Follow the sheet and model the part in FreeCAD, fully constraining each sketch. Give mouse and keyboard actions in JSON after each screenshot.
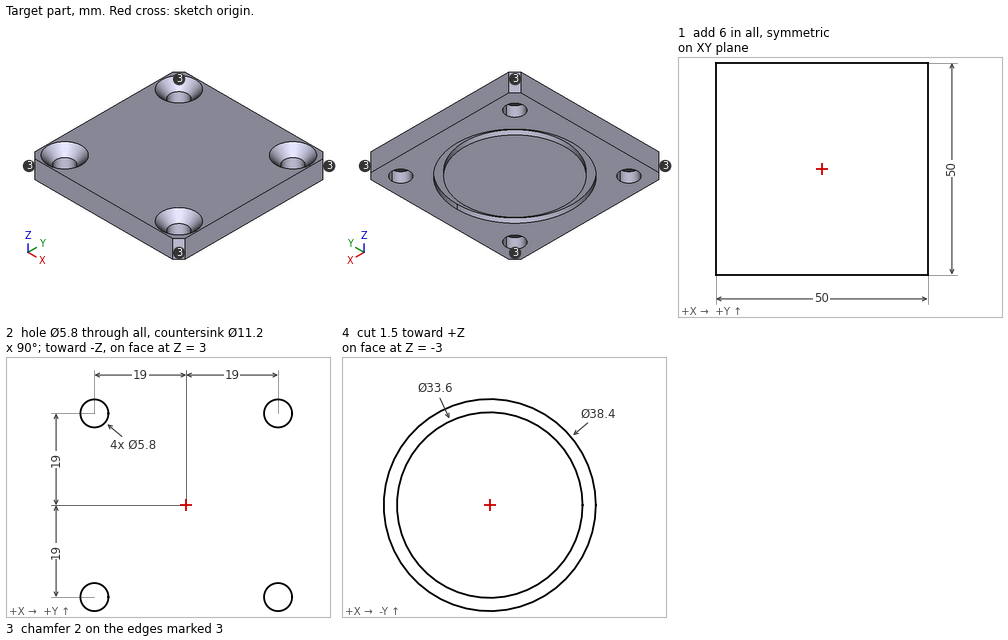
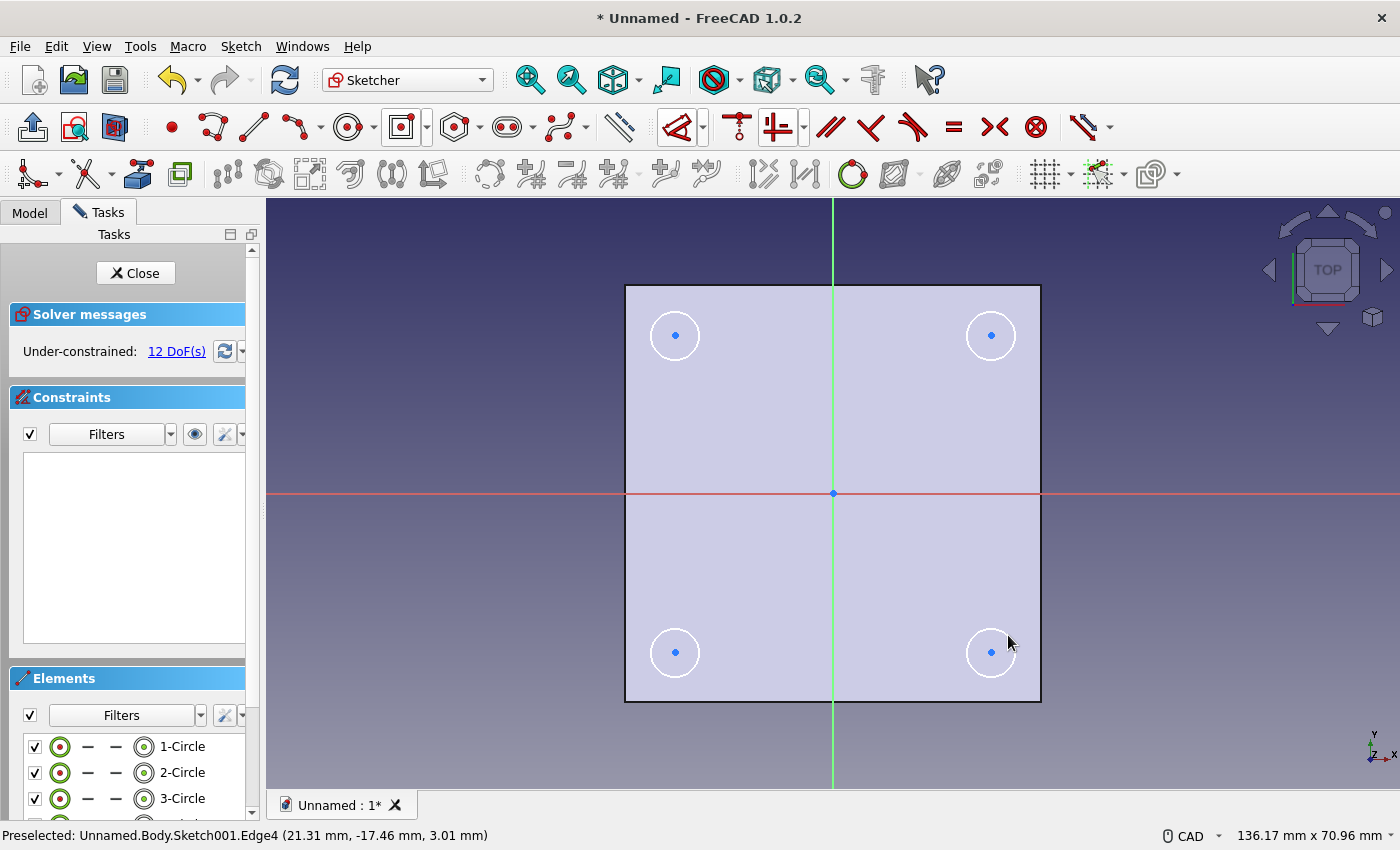
{"action": "left_click", "coordinate": [692, 319]}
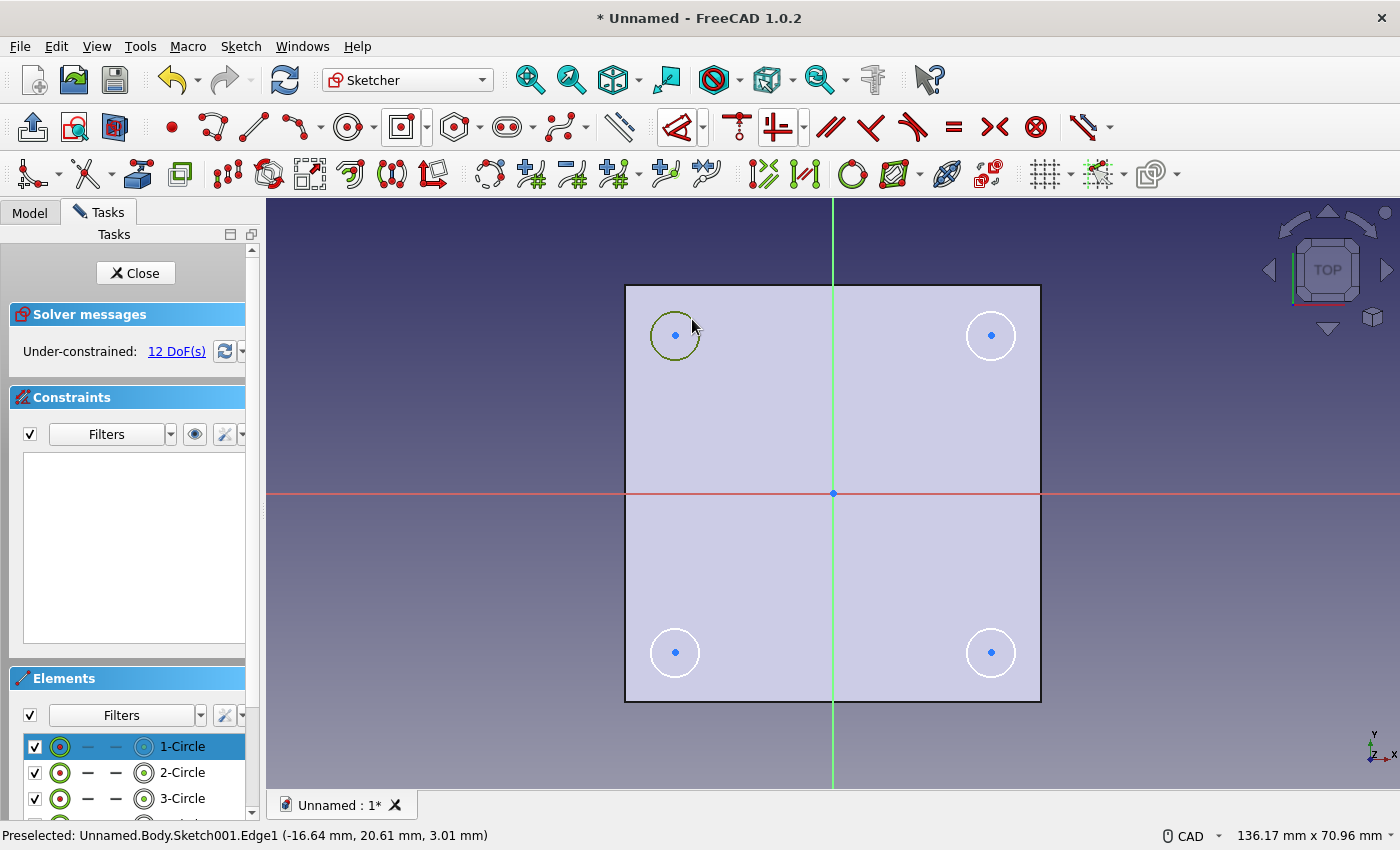
{"action": "left_click", "coordinate": [1008, 319]}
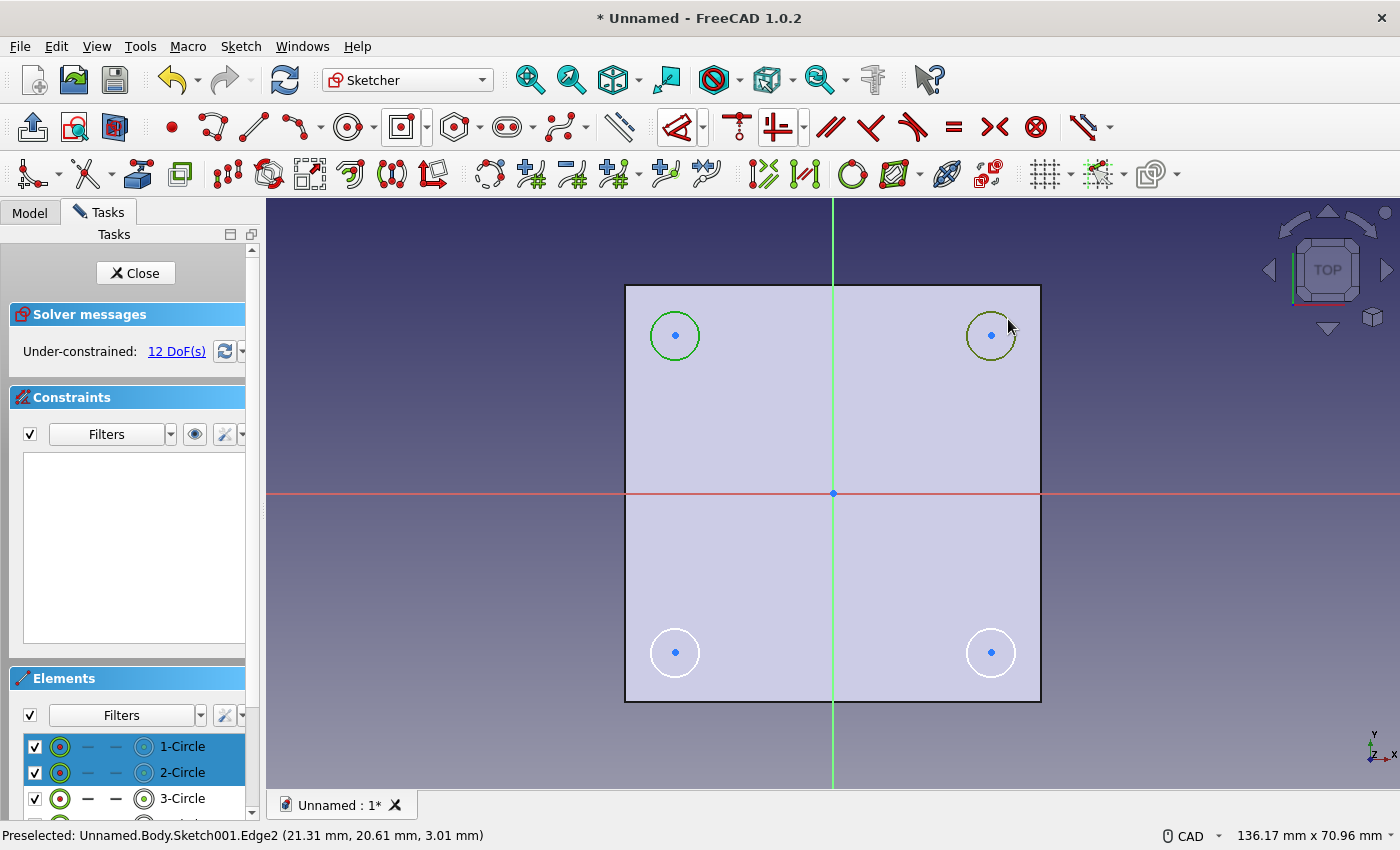
{"action": "left_click", "coordinate": [692, 636]}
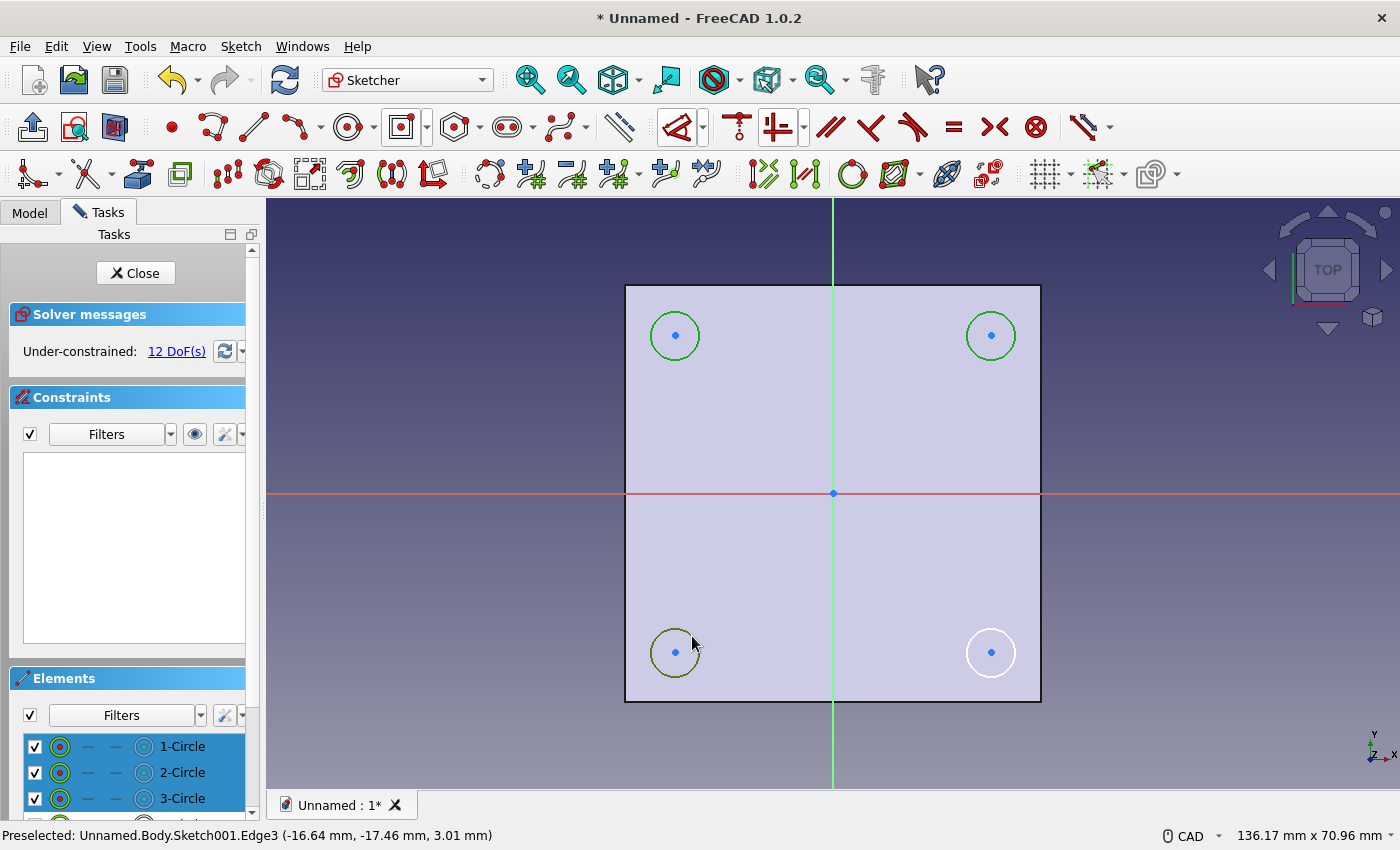
{"action": "left_click", "coordinate": [1008, 636]}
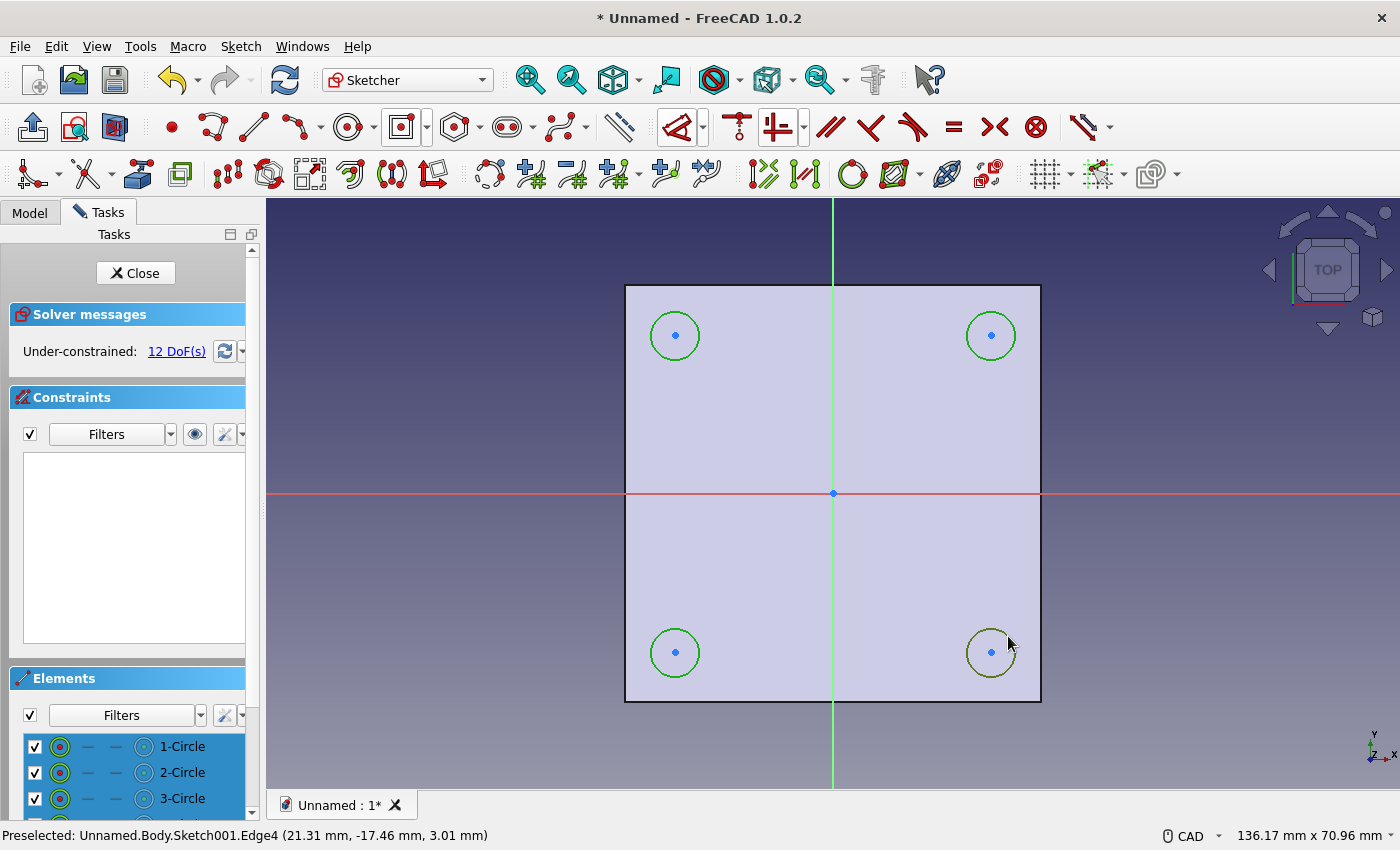
{"action": "left_click", "coordinate": [954, 128]}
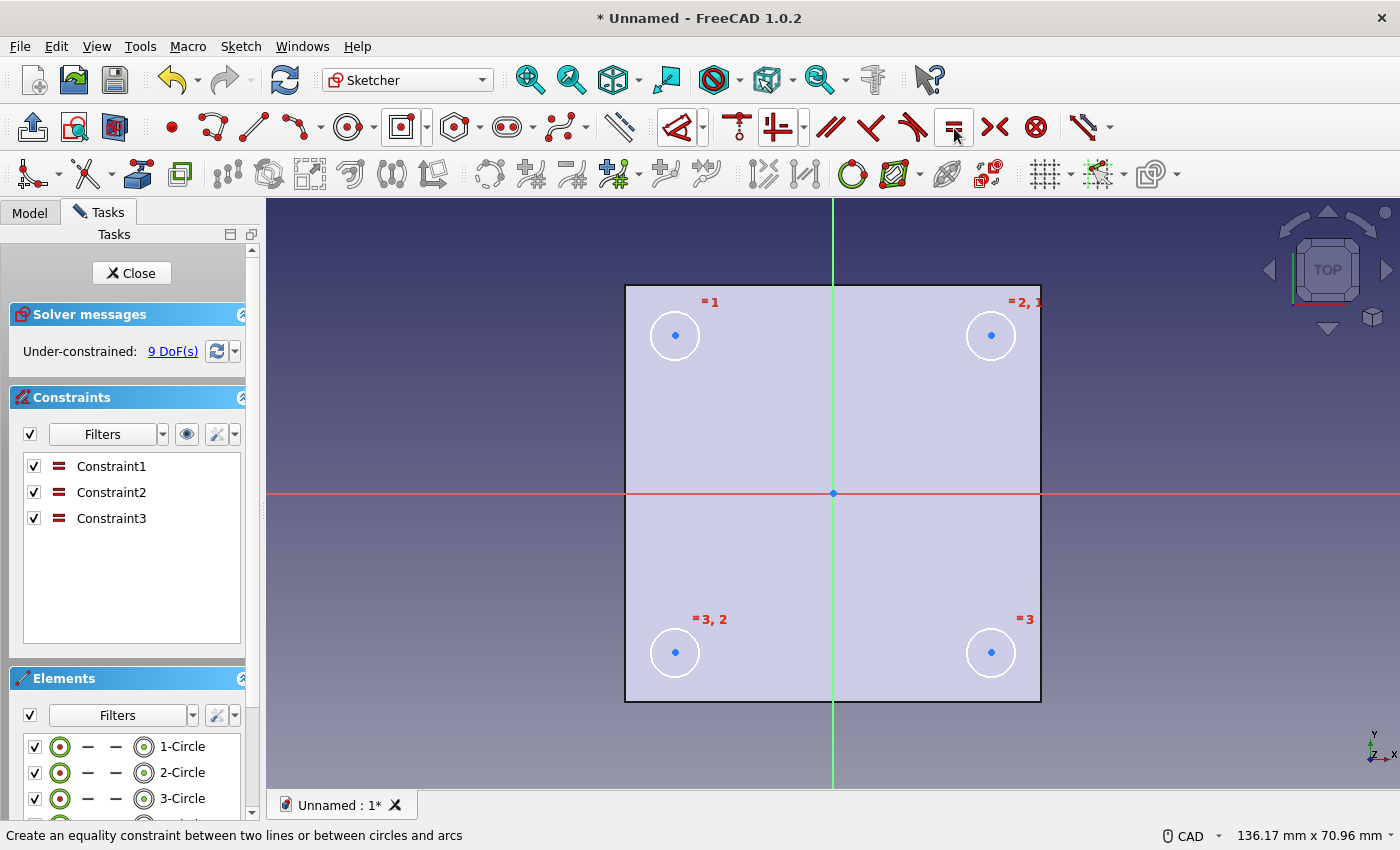
{"action": "left_click", "coordinate": [675, 336]}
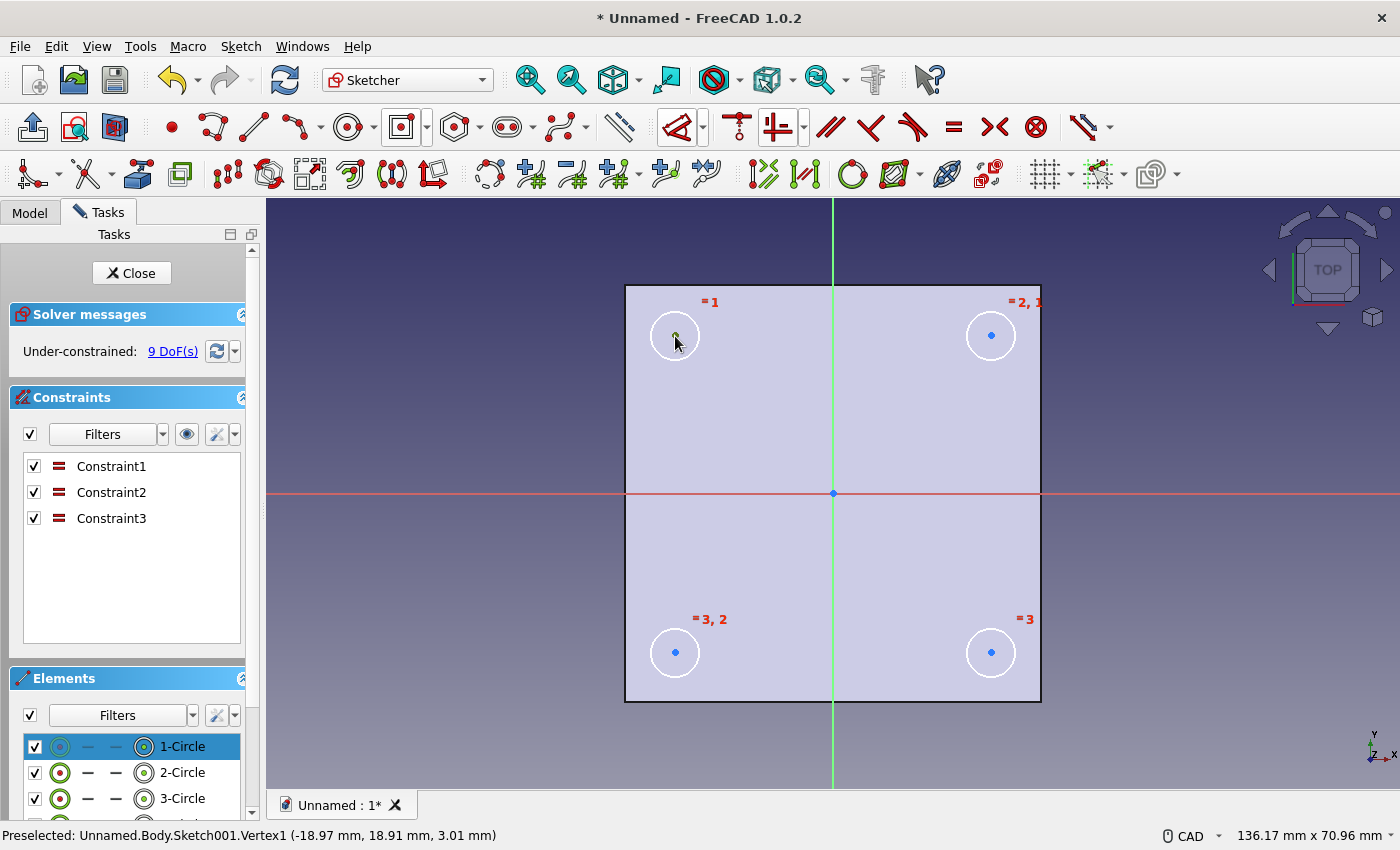
{"action": "left_click", "coordinate": [991, 336]}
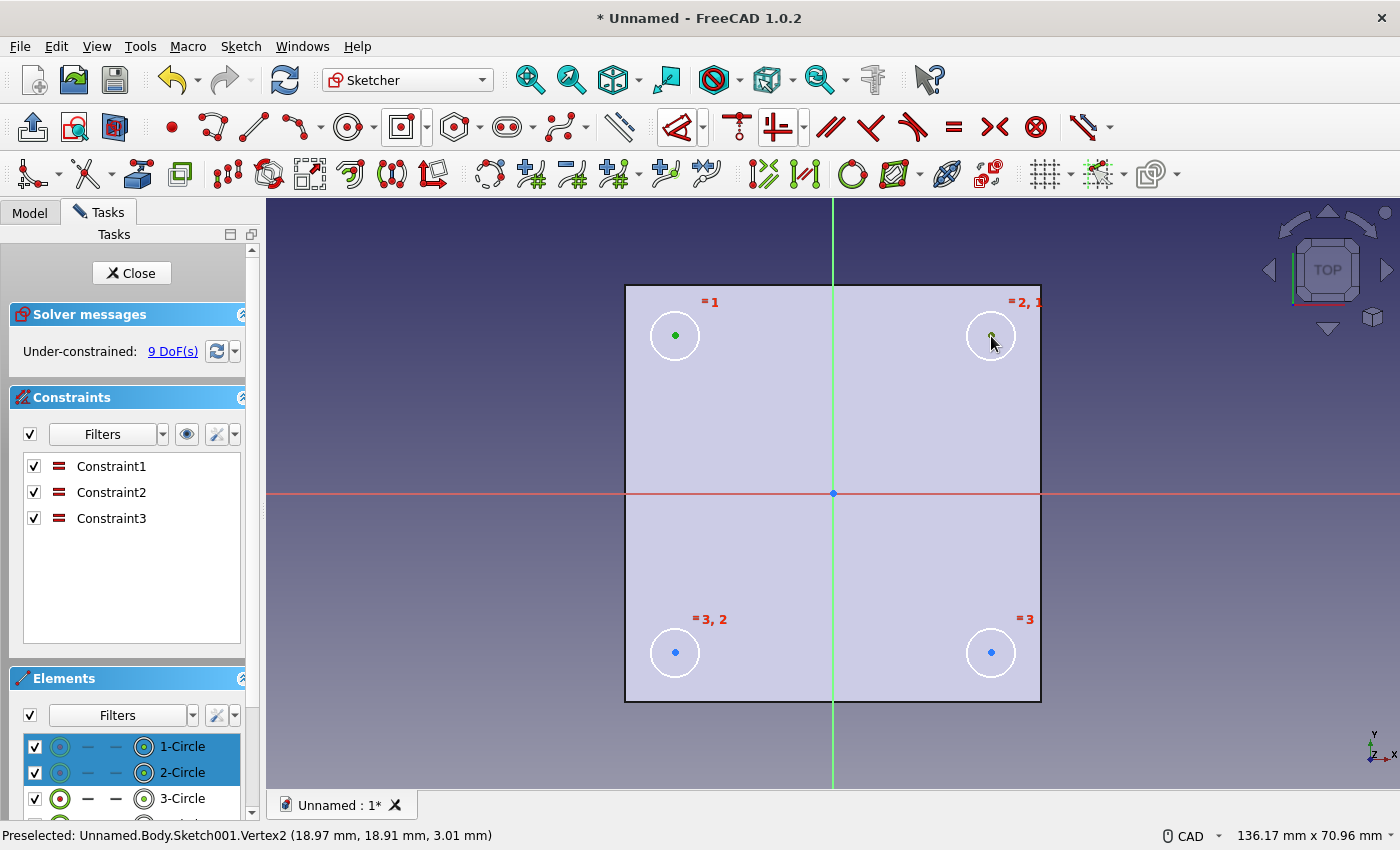
{"action": "left_click", "coordinate": [804, 128]}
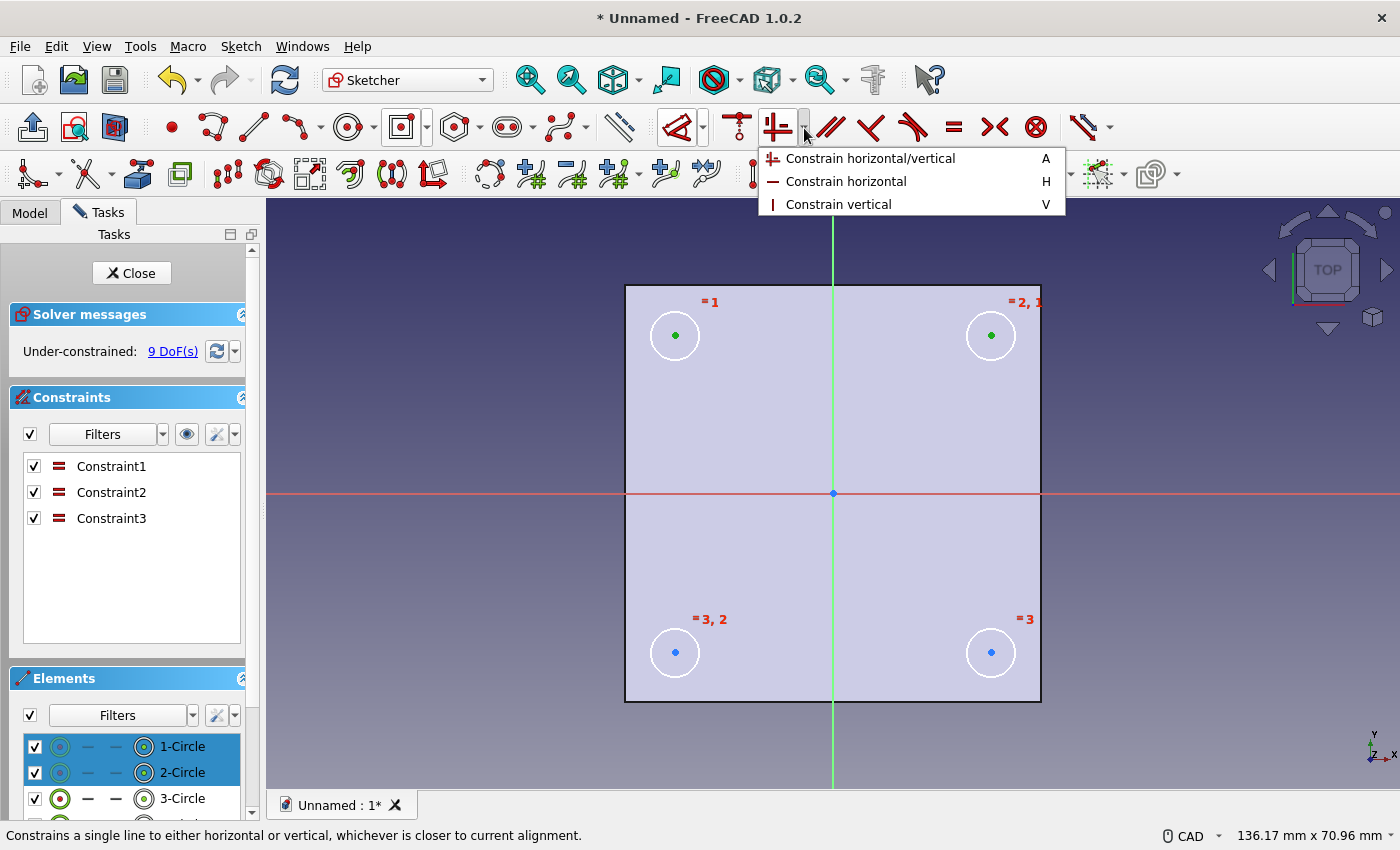
{"action": "left_click", "coordinate": [912, 182]}